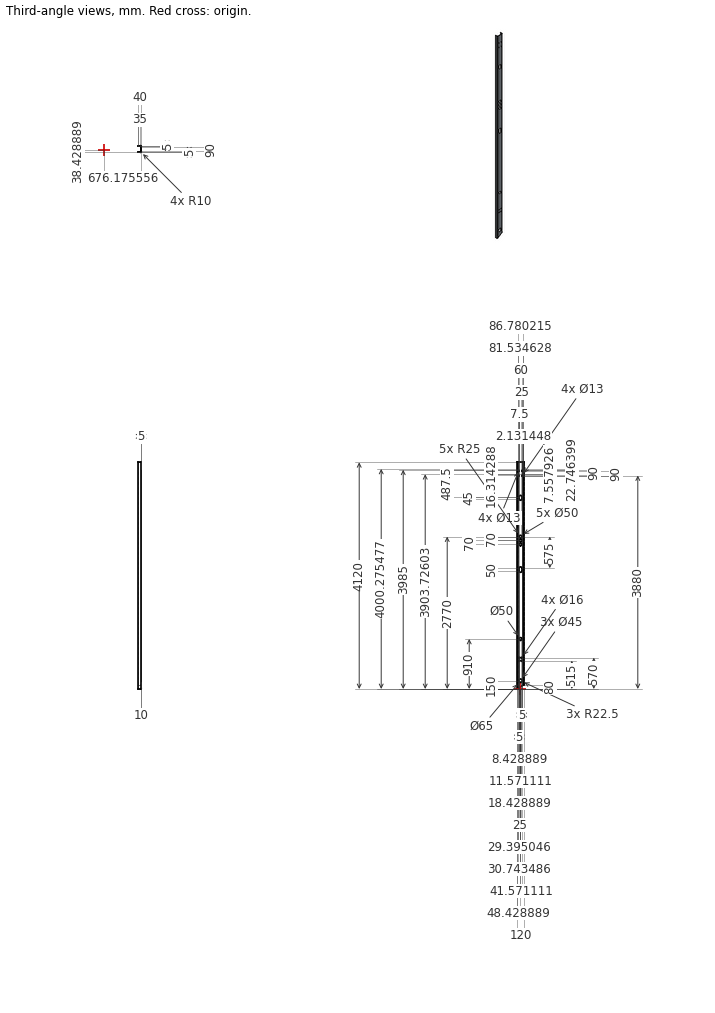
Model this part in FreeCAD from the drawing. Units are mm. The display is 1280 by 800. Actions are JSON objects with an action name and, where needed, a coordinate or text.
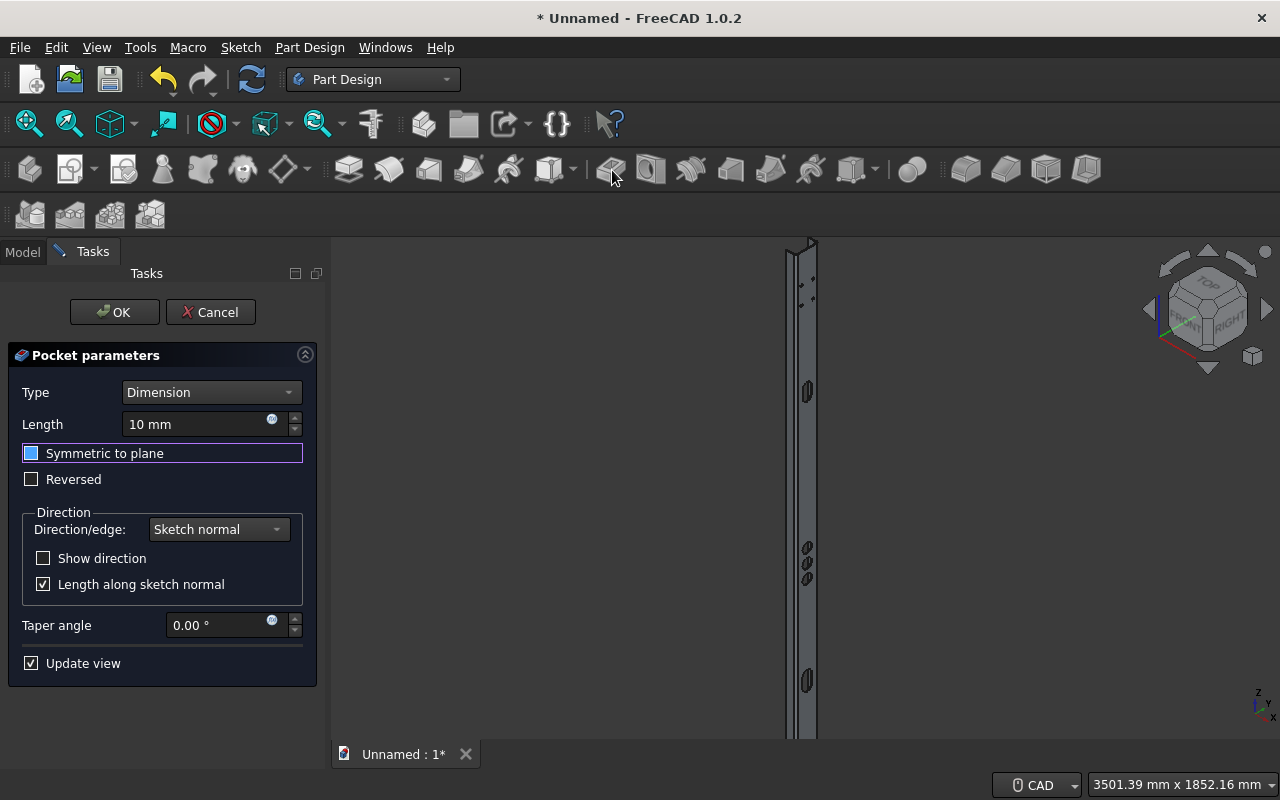
{"action": "left_click", "coordinate": [115, 312]}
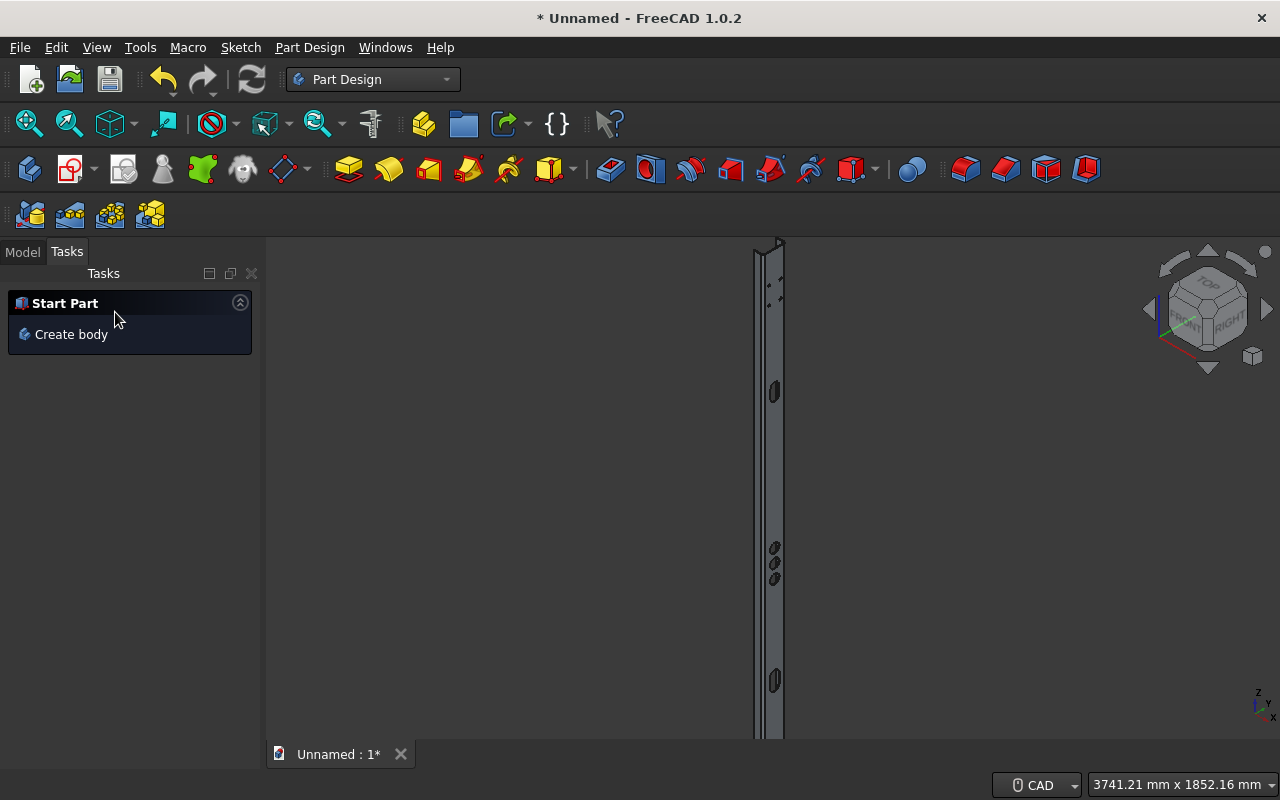
{"action": "left_click", "coordinate": [30, 124]}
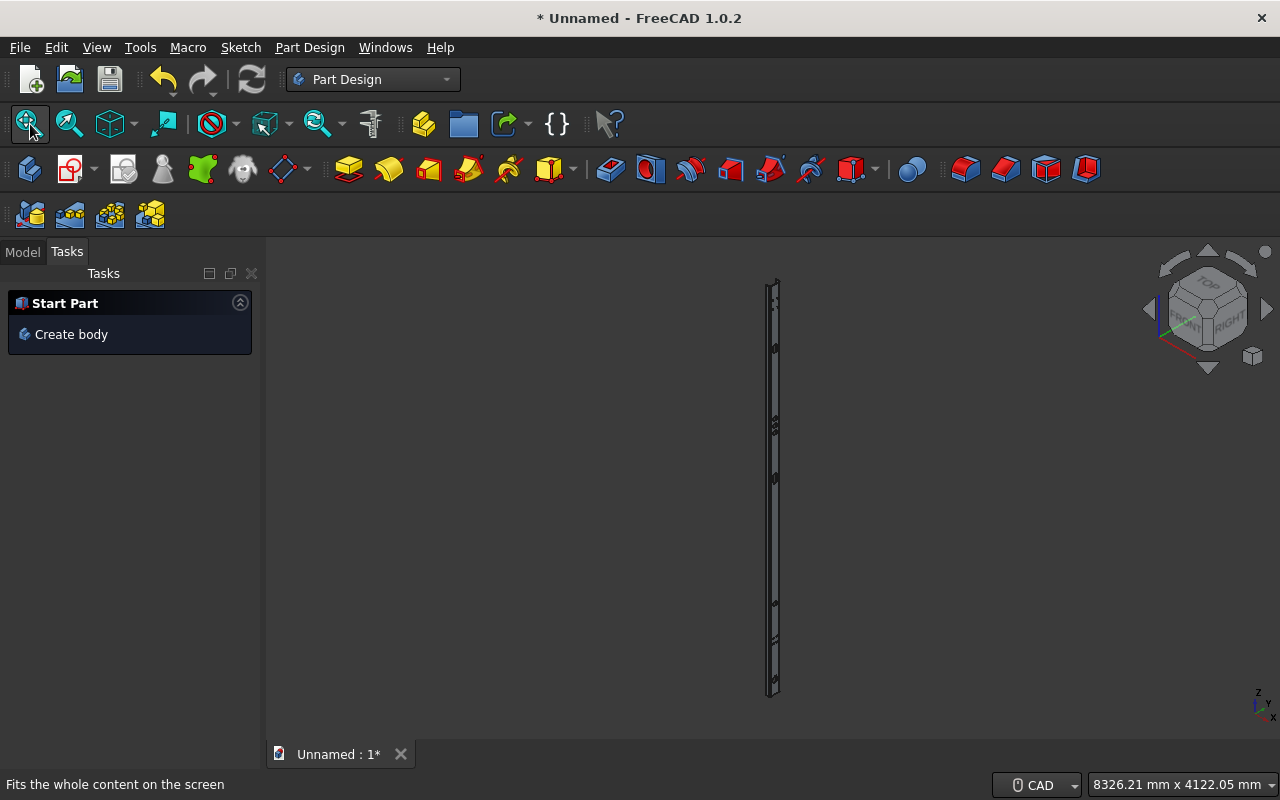
{"action": "scroll", "coordinate": [775, 313], "scroll_direction": "up", "scroll_amount": 4}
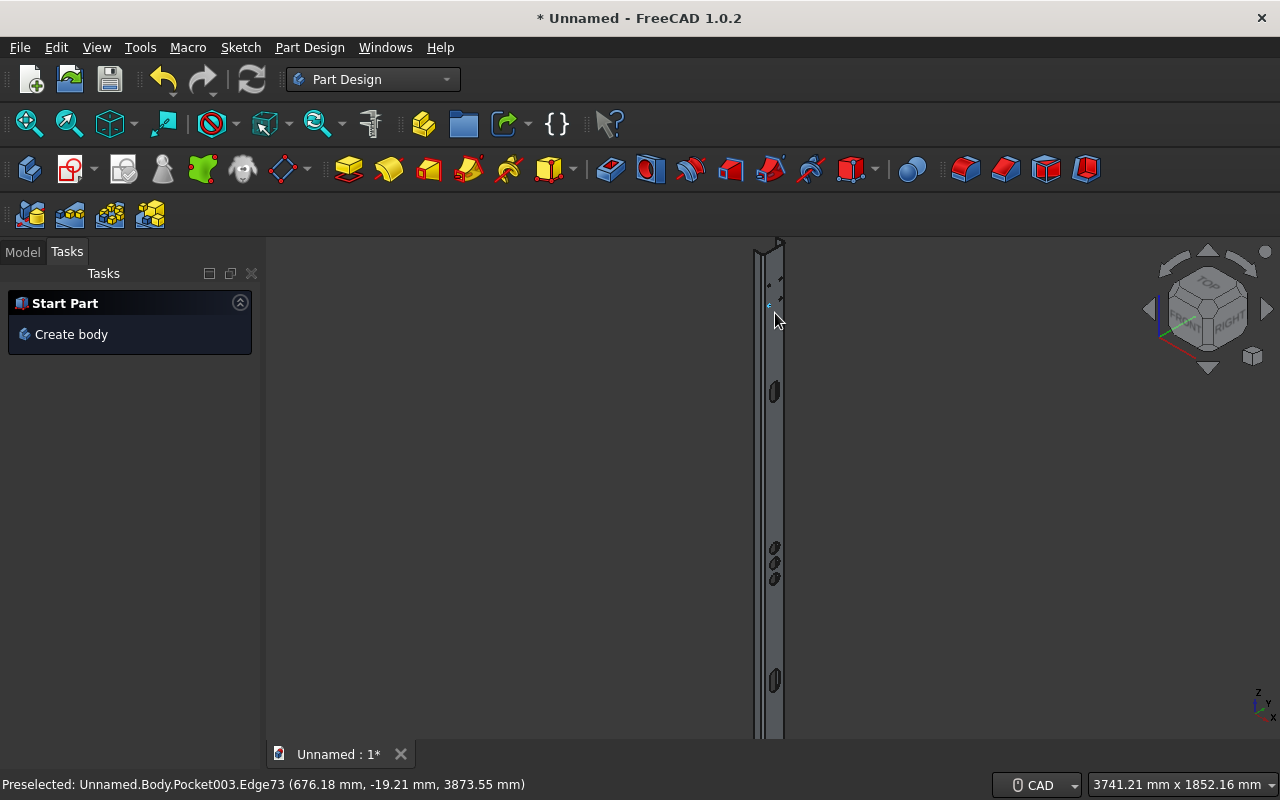
{"action": "left_click", "coordinate": [775, 444]}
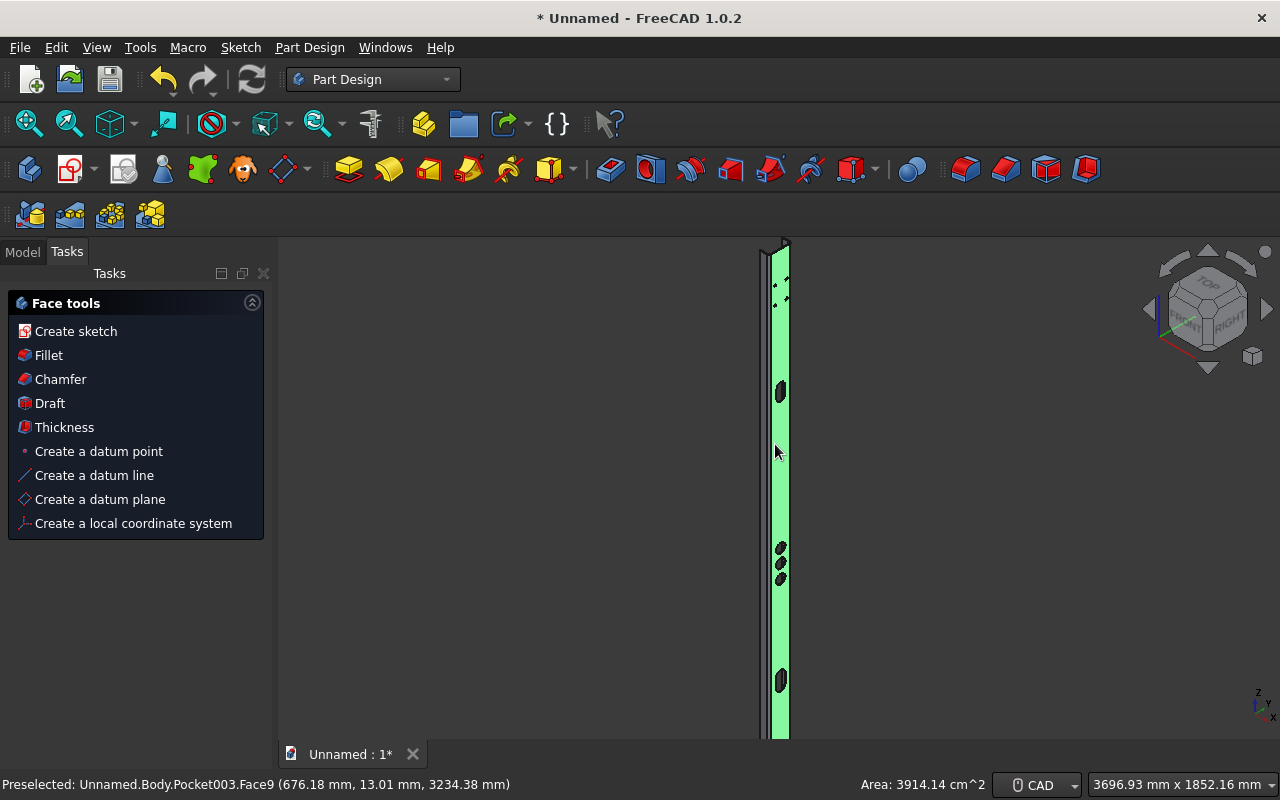
{"action": "left_click", "coordinate": [70, 170]}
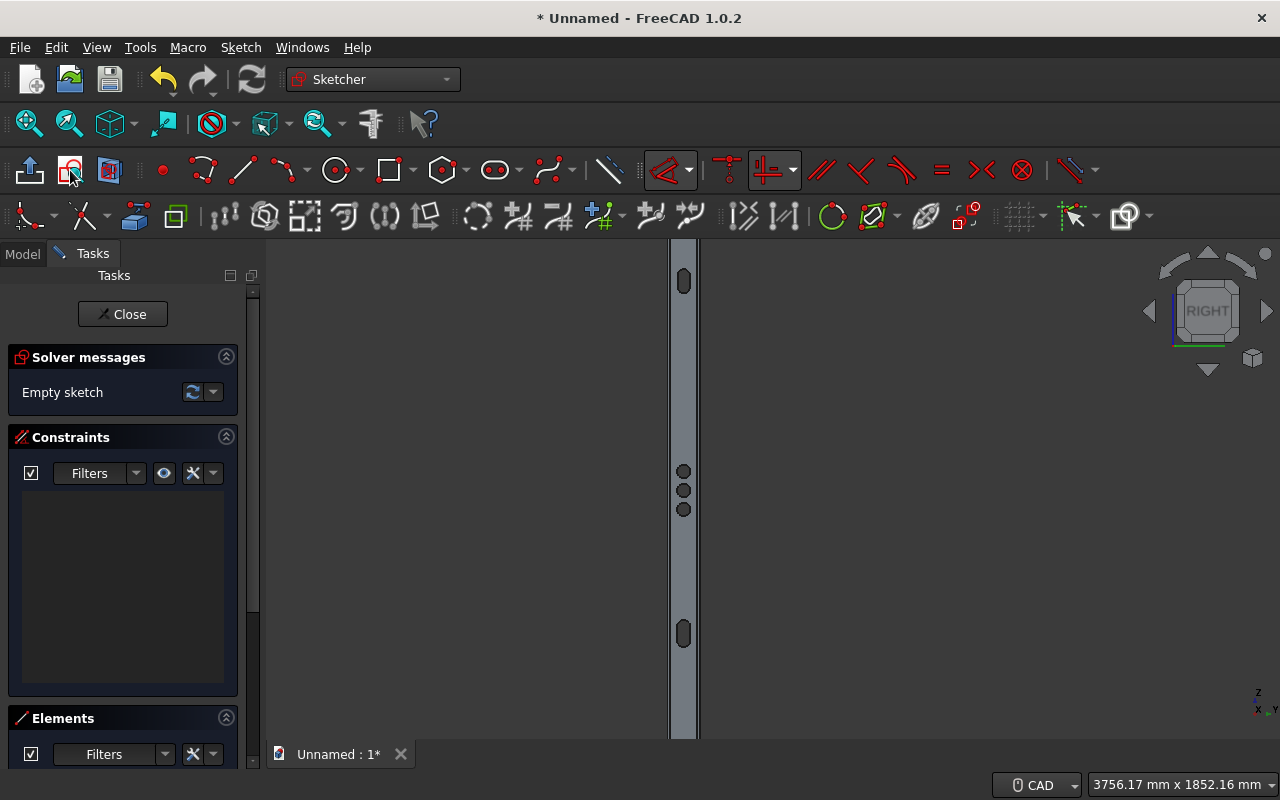
{"action": "scroll", "coordinate": [704, 489], "scroll_direction": "down", "scroll_amount": 5}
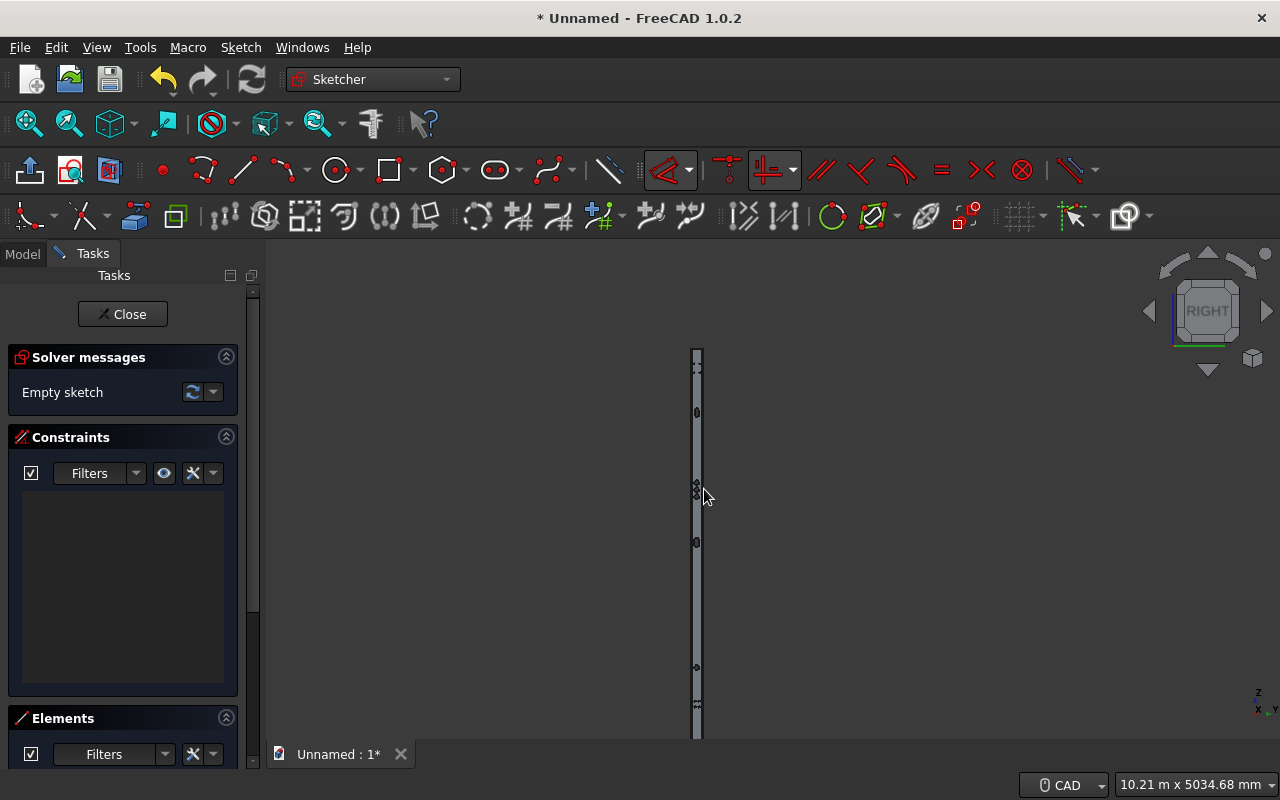
{"action": "scroll", "coordinate": [704, 489], "scroll_direction": "down", "scroll_amount": 5}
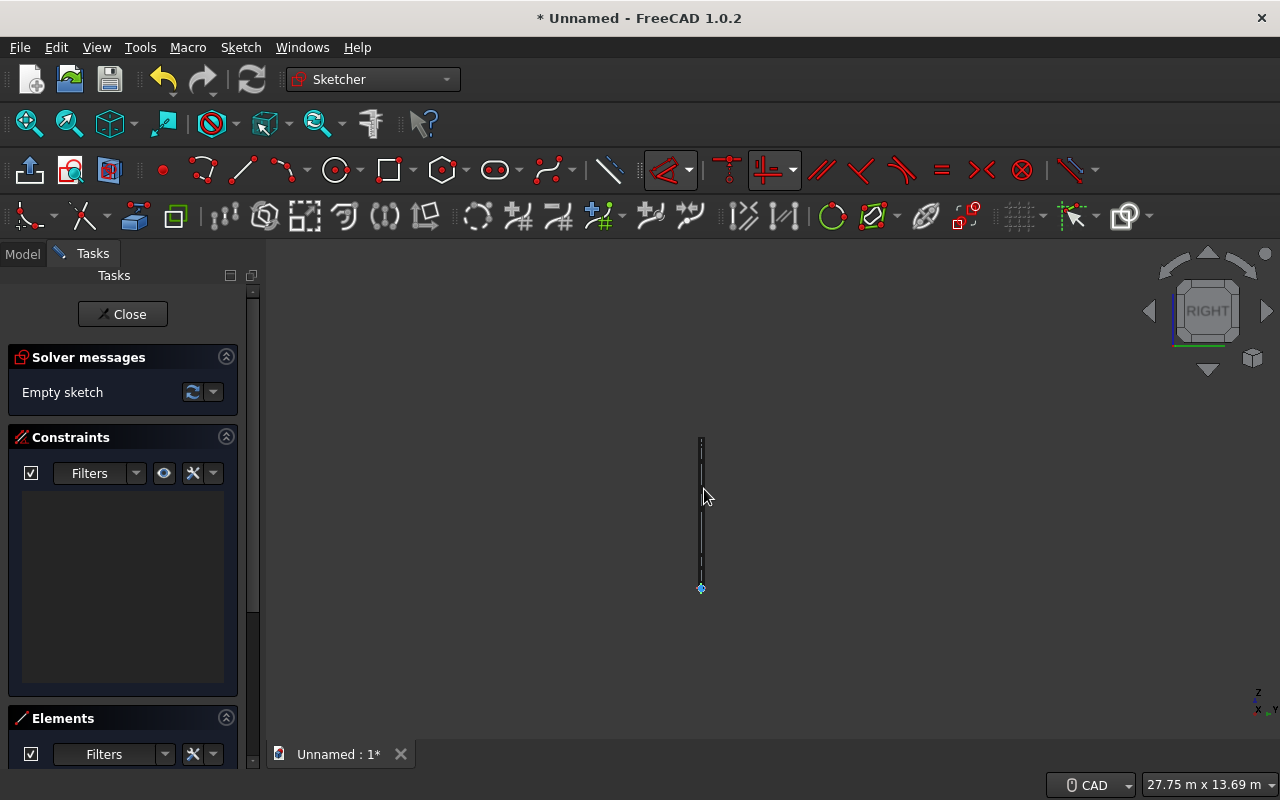
{"action": "scroll", "coordinate": [701, 592], "scroll_direction": "up", "scroll_amount": 15}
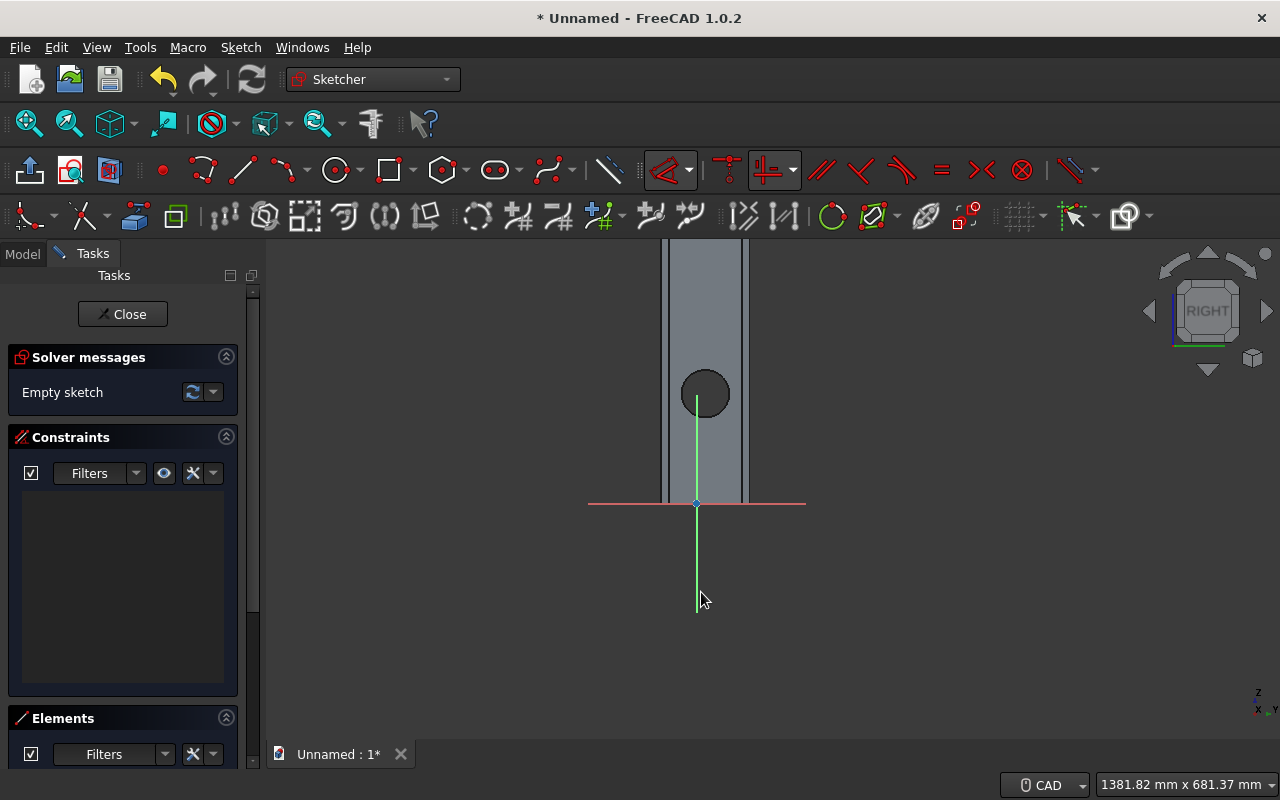
{"action": "scroll", "coordinate": [706, 471], "scroll_direction": "up", "scroll_amount": 8}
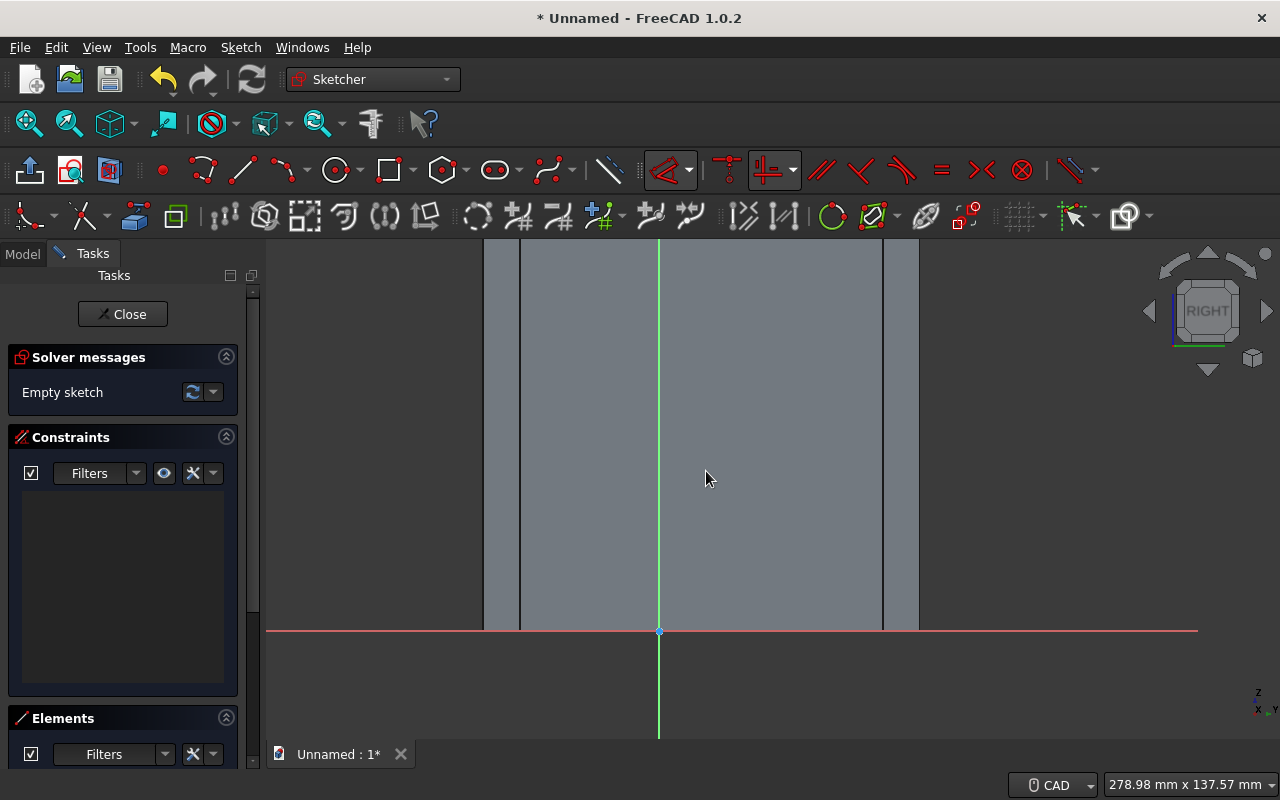
{"action": "left_click", "coordinate": [204, 170]}